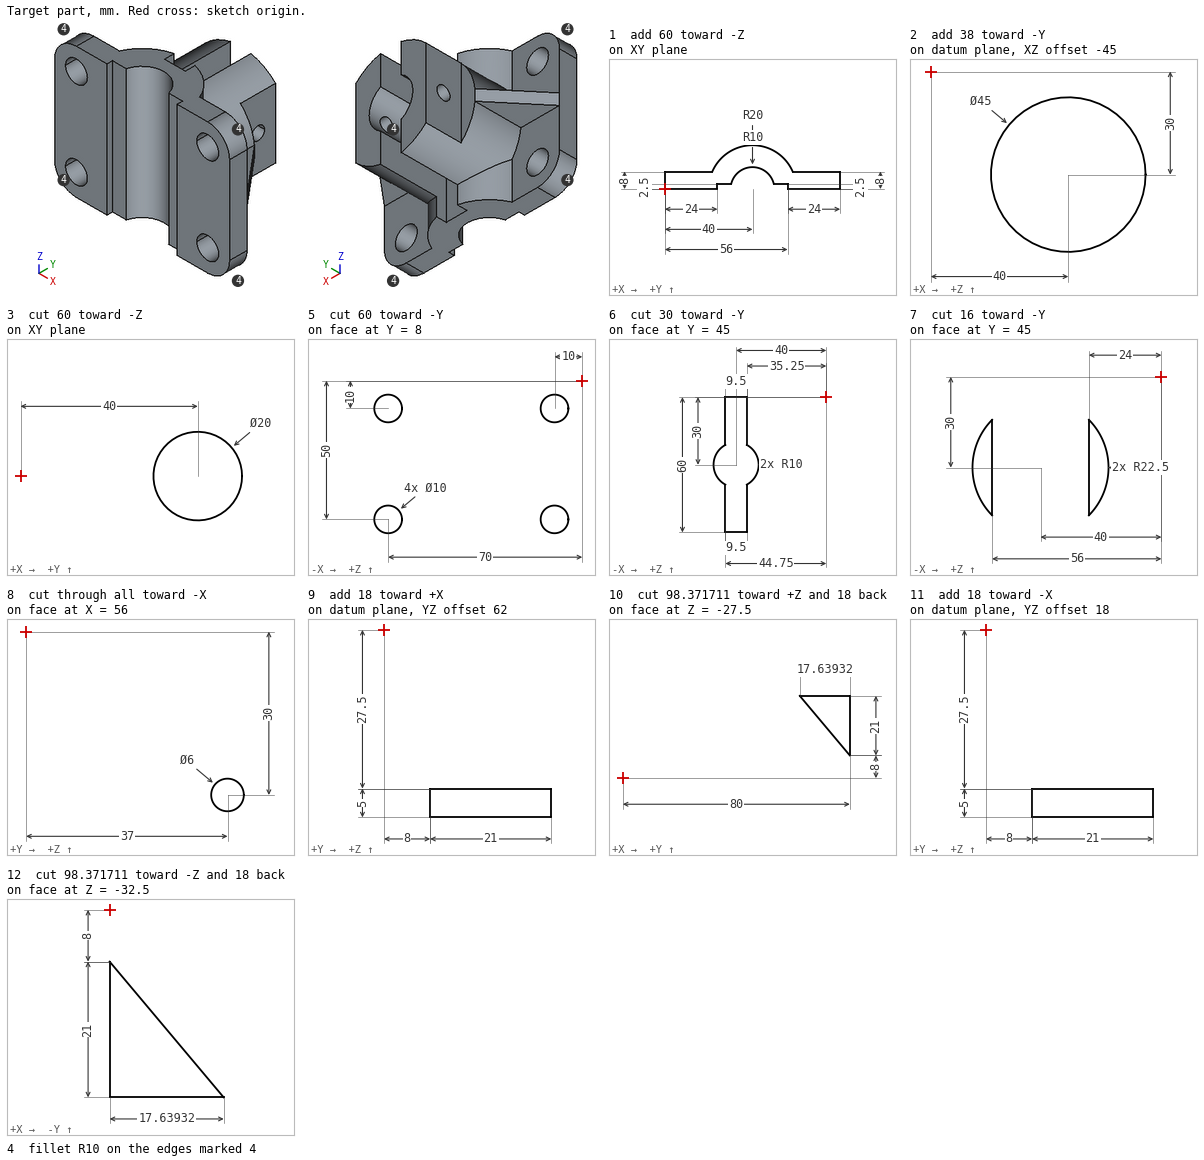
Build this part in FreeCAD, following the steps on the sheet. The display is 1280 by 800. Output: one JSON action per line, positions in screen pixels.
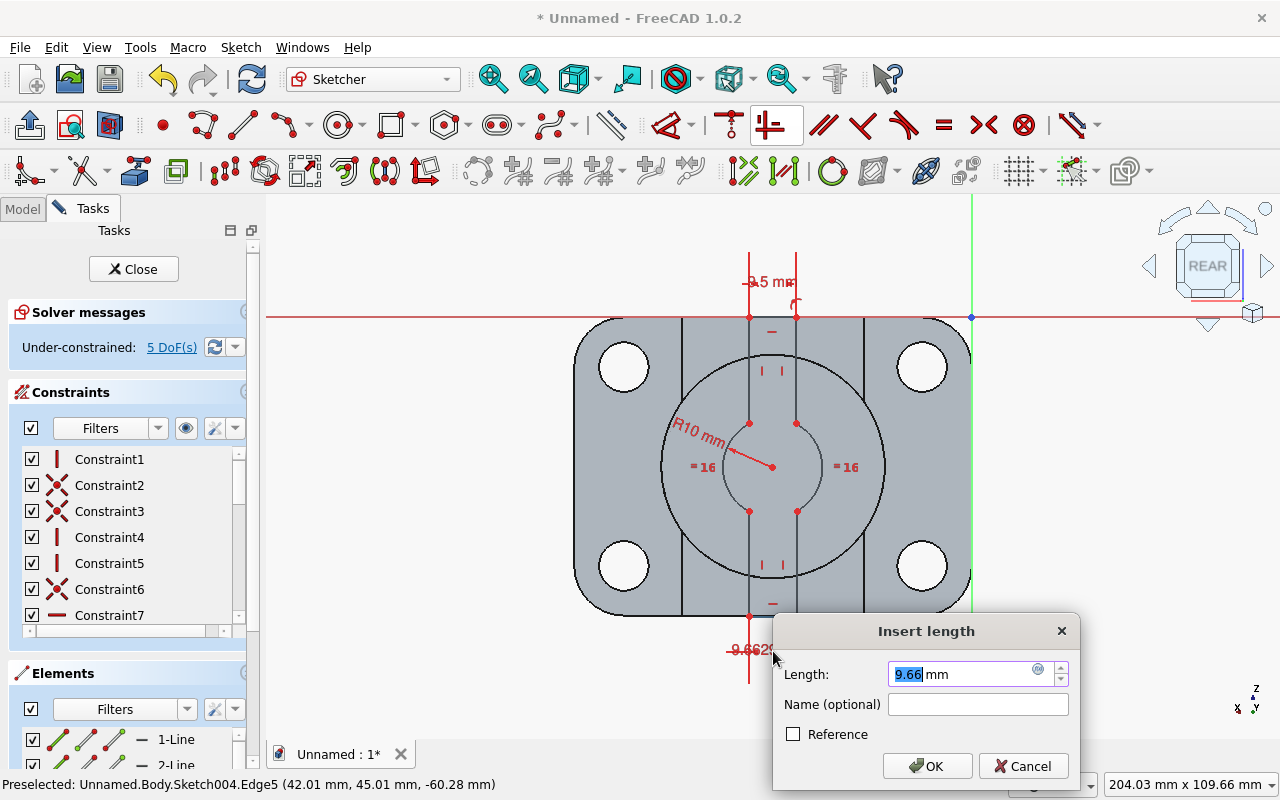
{"action": "type", "text": "9.5"}
{"action": "key", "text": "Return"}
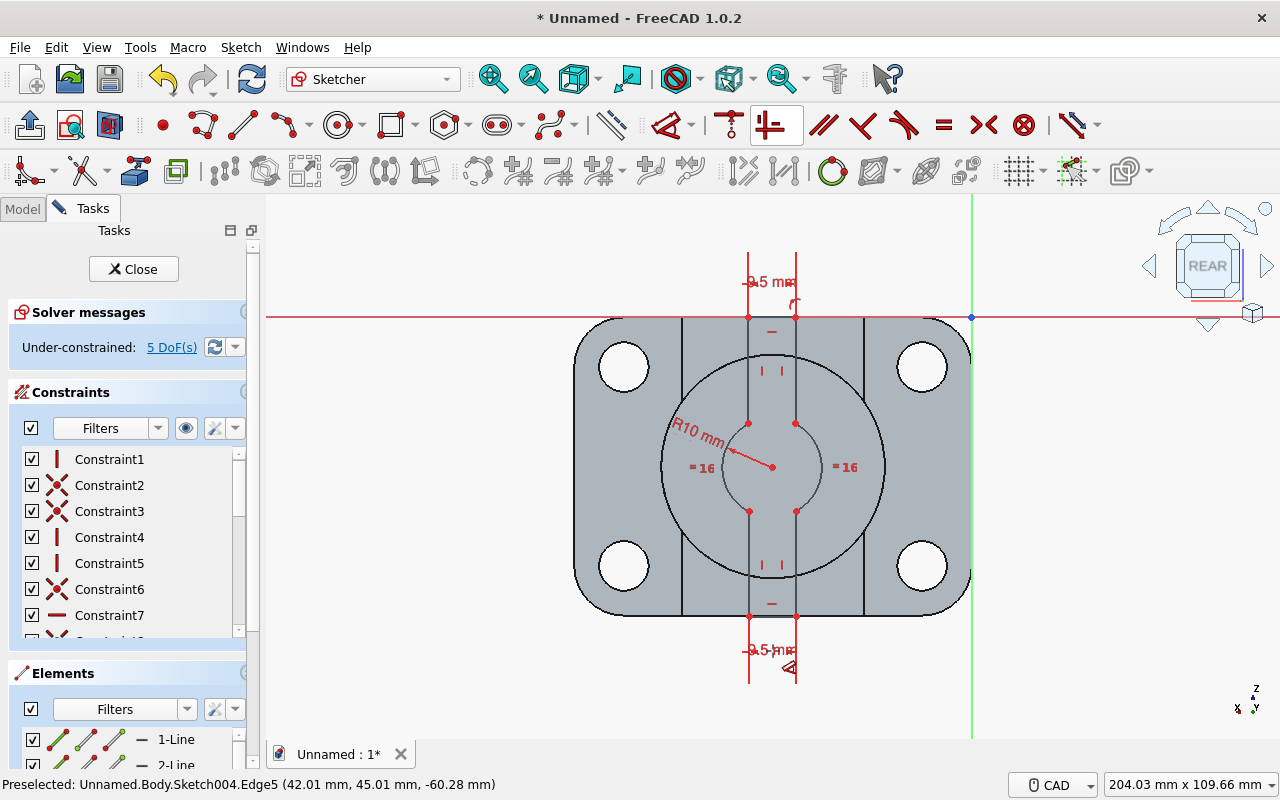
{"action": "left_click", "coordinate": [749, 617]}
{"action": "left_click", "coordinate": [1006, 467]}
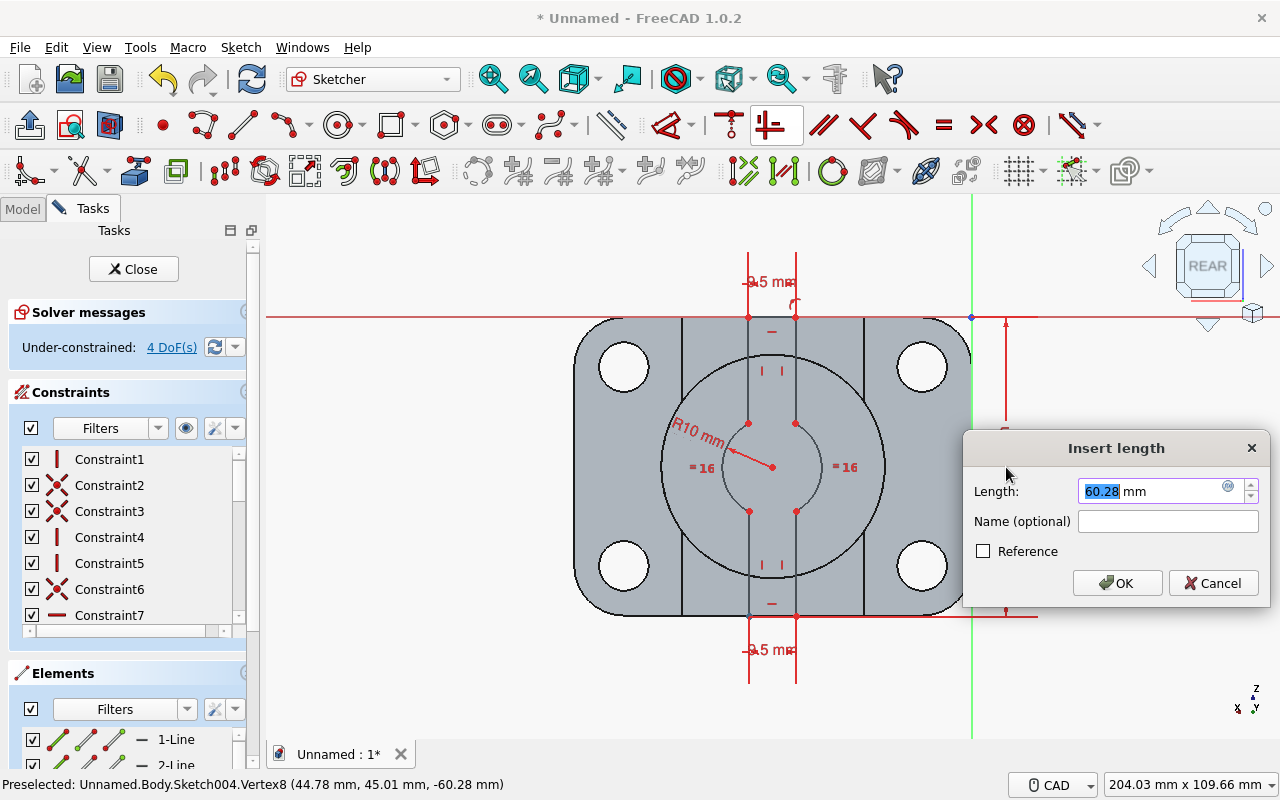
{"action": "type", "text": "60"}
{"action": "key", "text": "Return"}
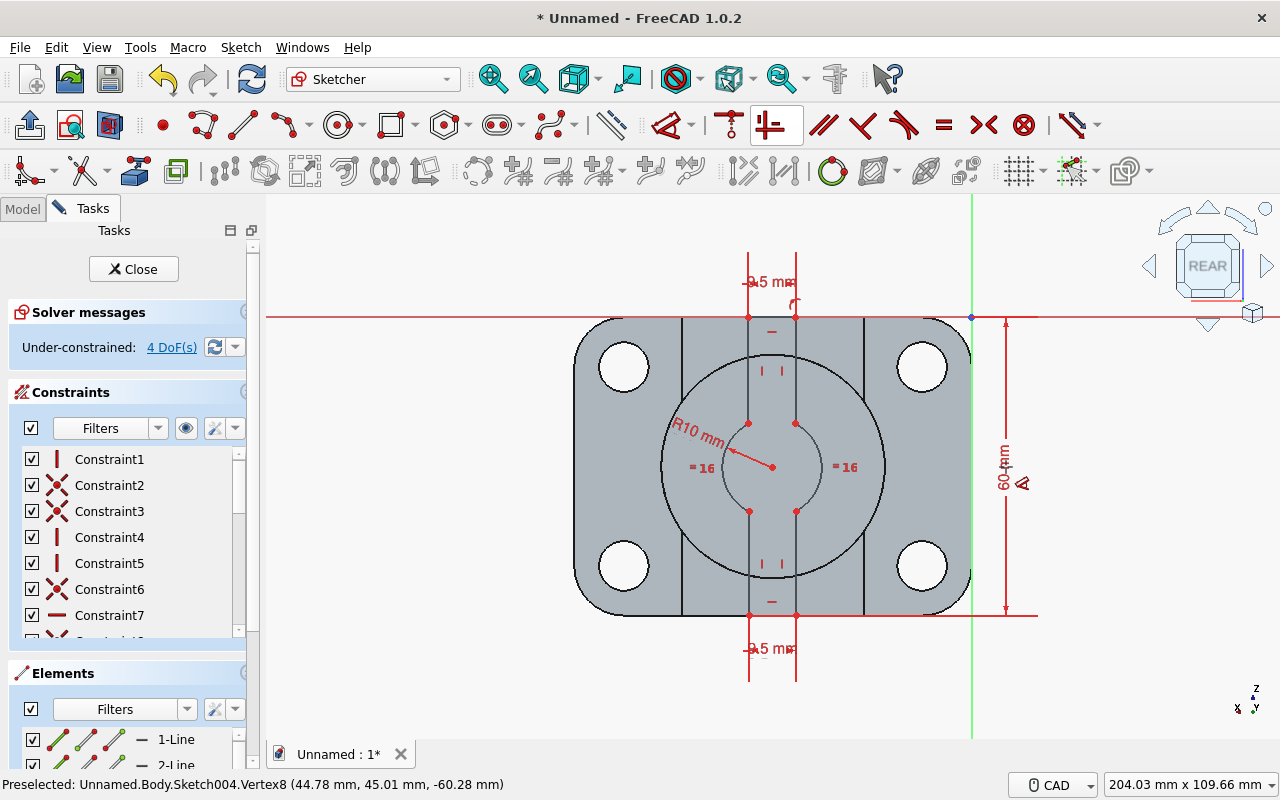
{"action": "left_click", "coordinate": [772, 468]}
{"action": "left_click", "coordinate": [872, 283]}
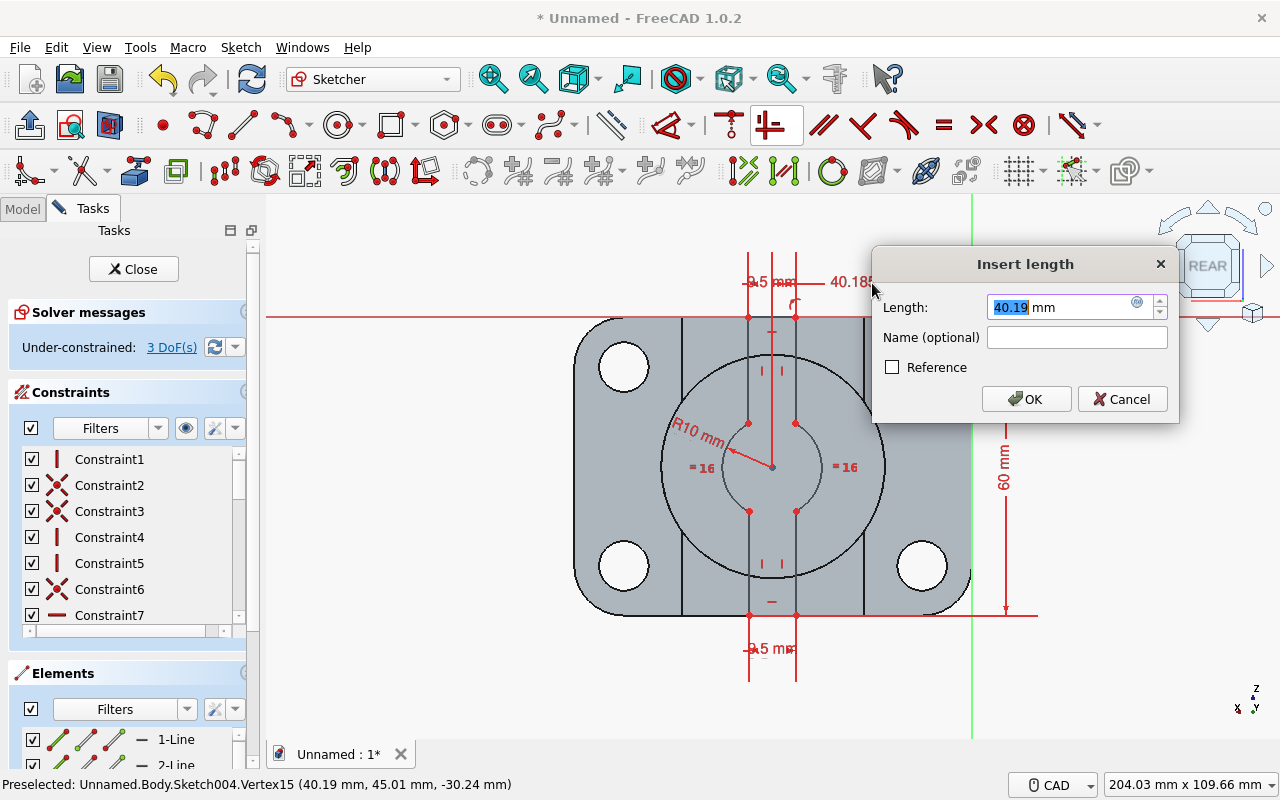
{"action": "type", "text": "40"}
{"action": "key", "text": "Return"}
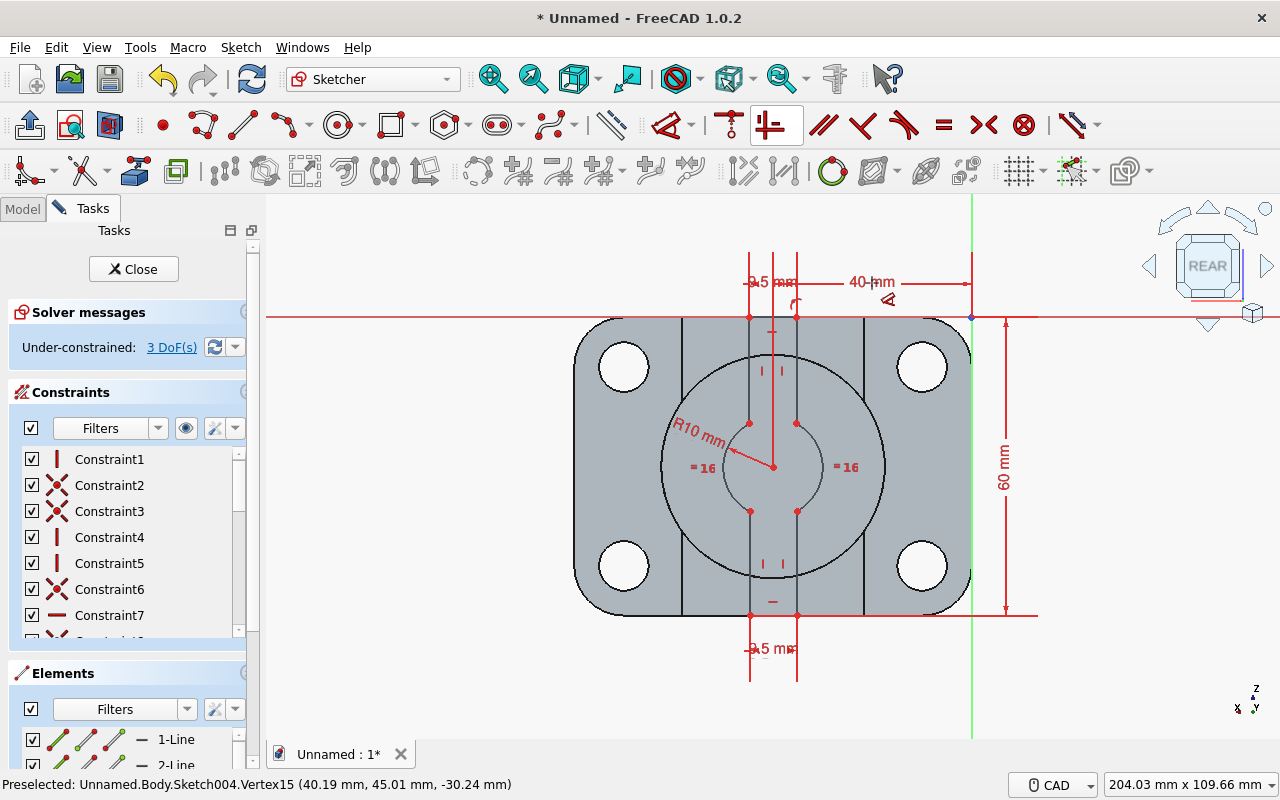
{"action": "left_click", "coordinate": [773, 468]}
{"action": "left_click", "coordinate": [1006, 393]}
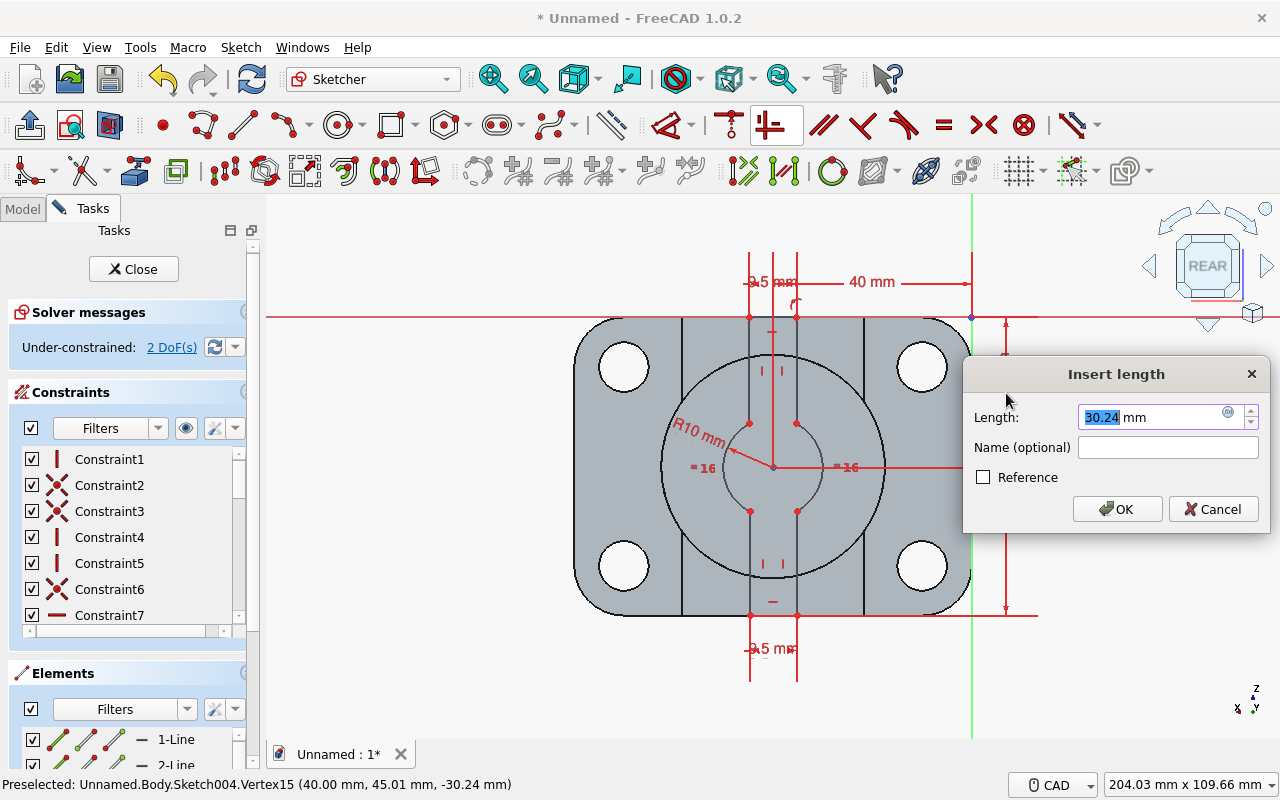
{"action": "type", "text": "30"}
{"action": "key", "text": "Return"}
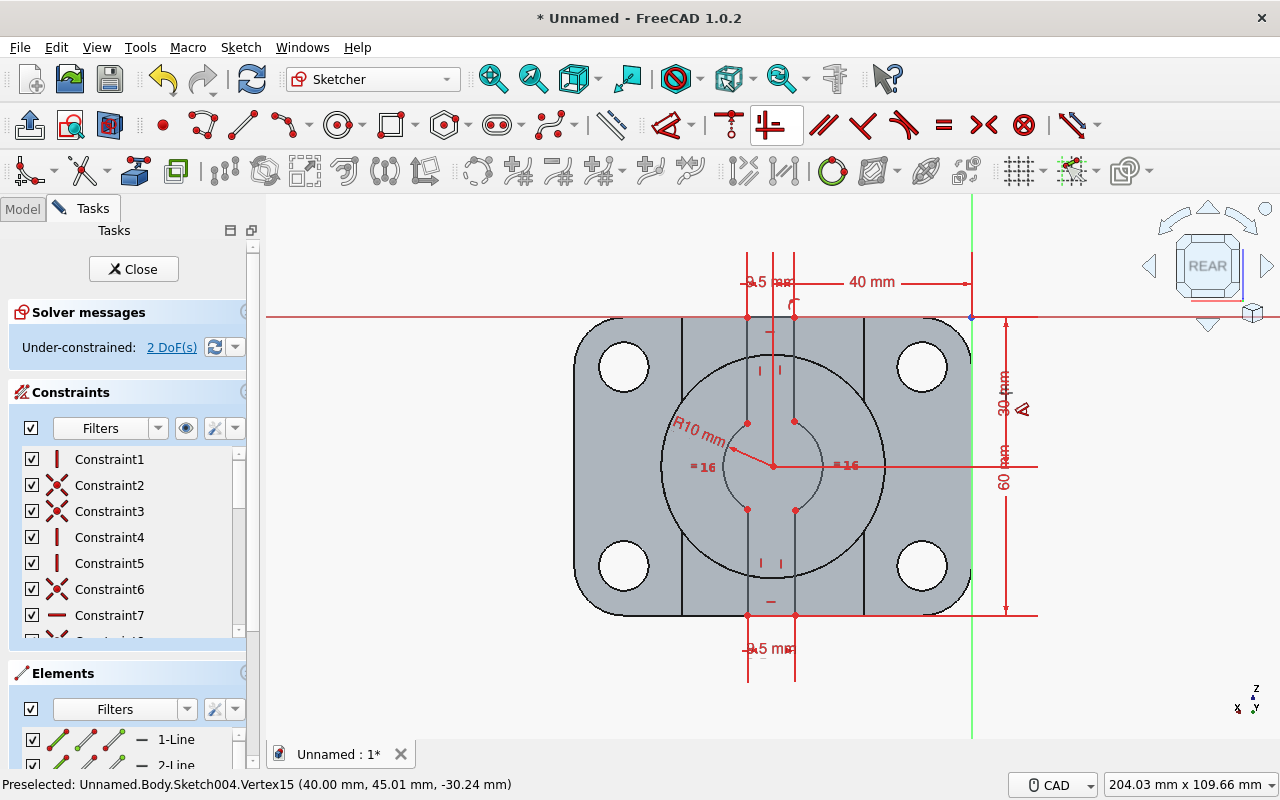
{"action": "left_click", "coordinate": [794, 422]}
{"action": "left_click", "coordinate": [945, 283]}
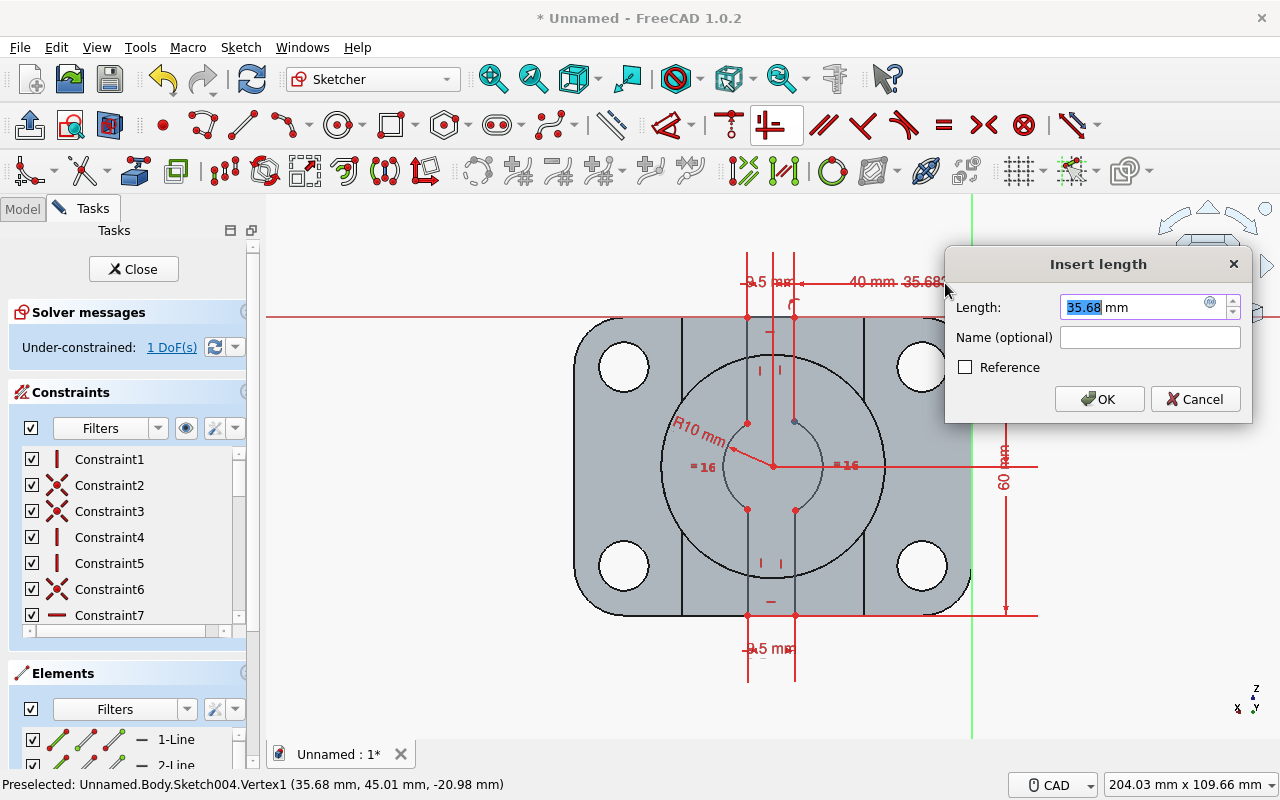
{"action": "type", "text": "35.25"}
{"action": "key", "text": "Return"}